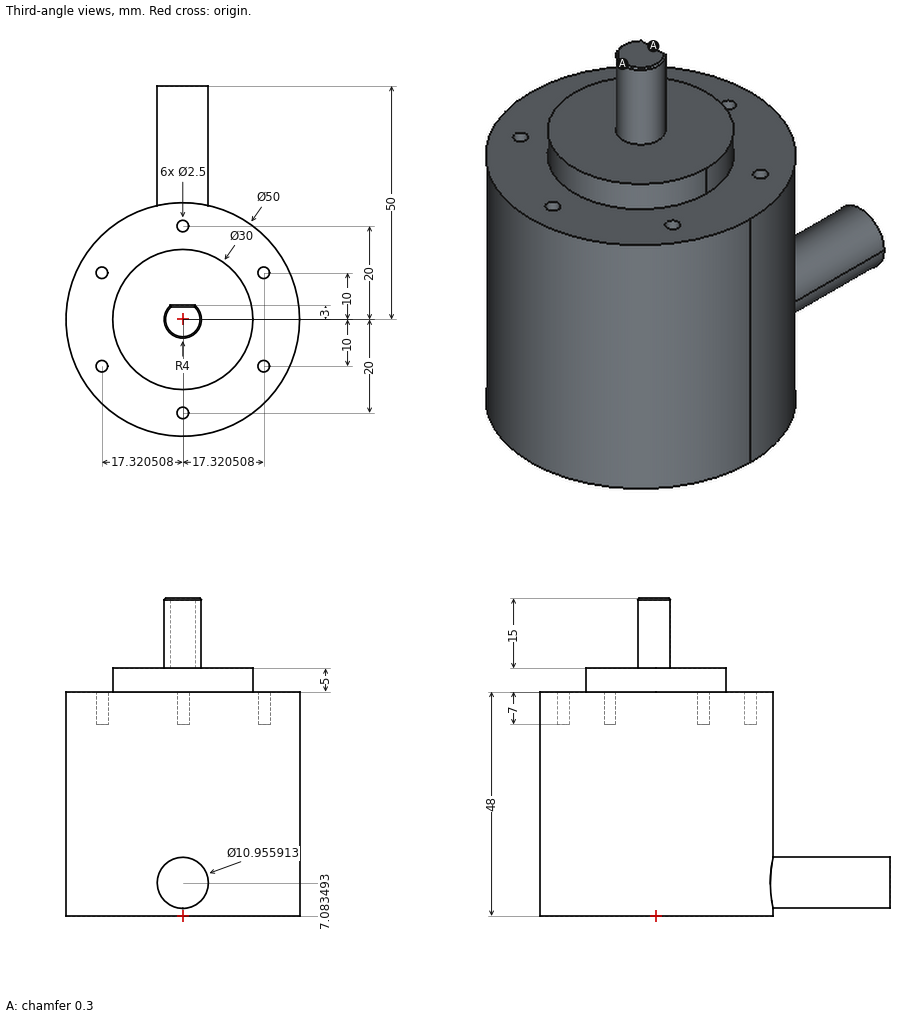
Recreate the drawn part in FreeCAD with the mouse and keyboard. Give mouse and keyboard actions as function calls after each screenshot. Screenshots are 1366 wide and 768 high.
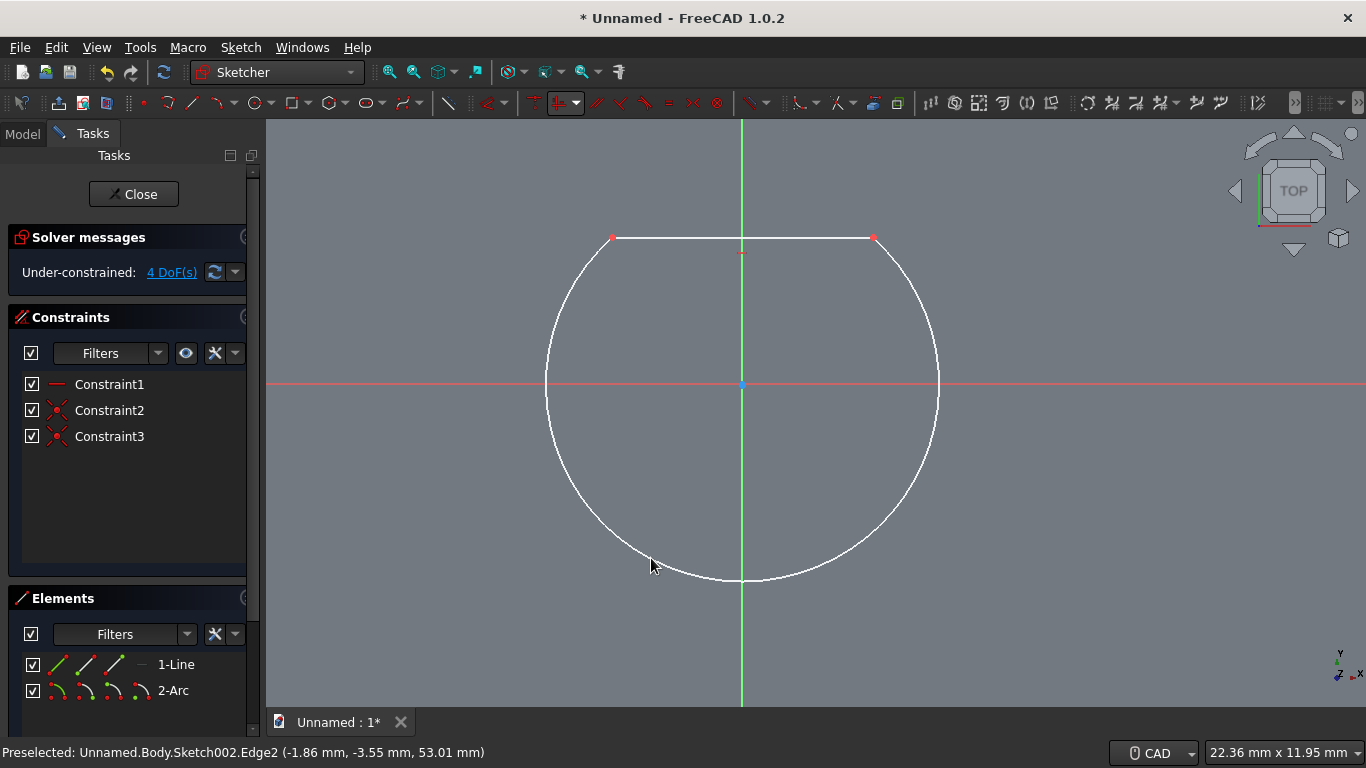
drag(732, 374, 752, 395)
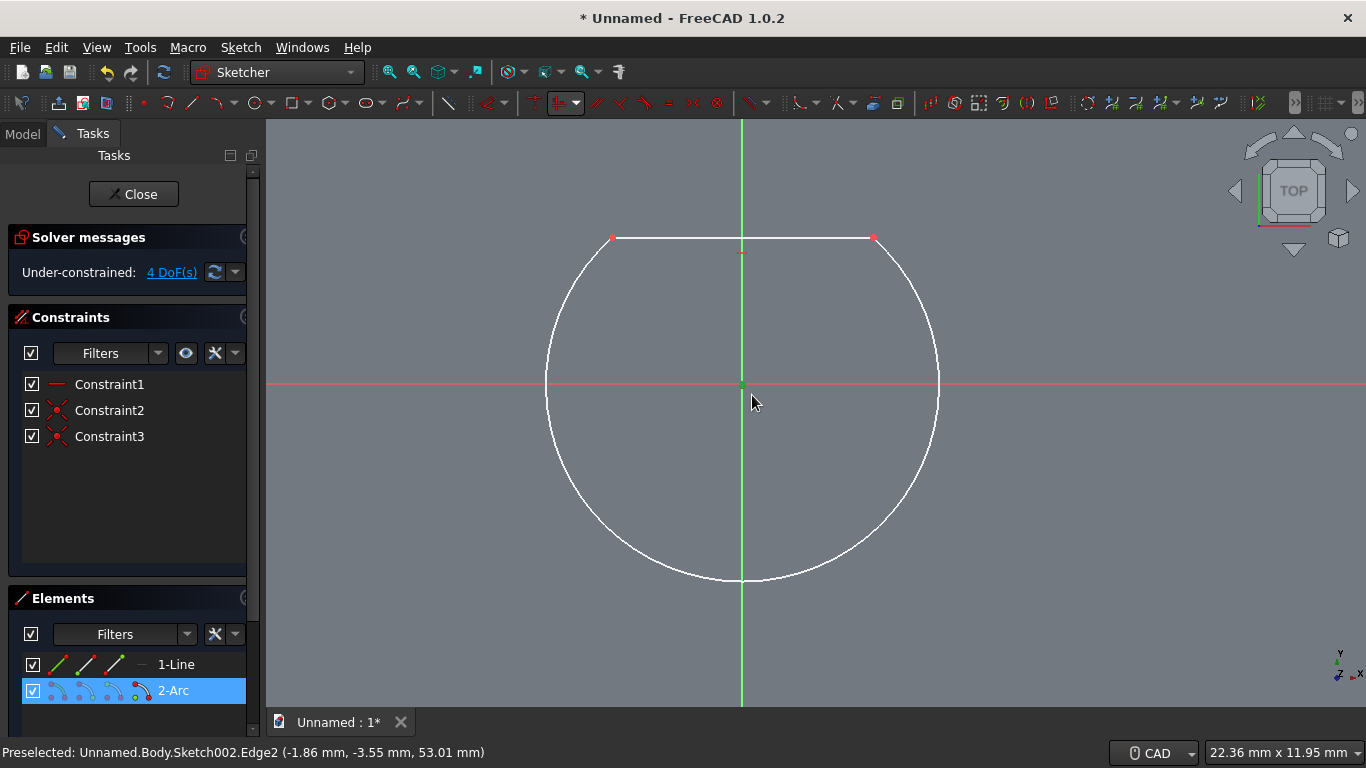
click(534, 104)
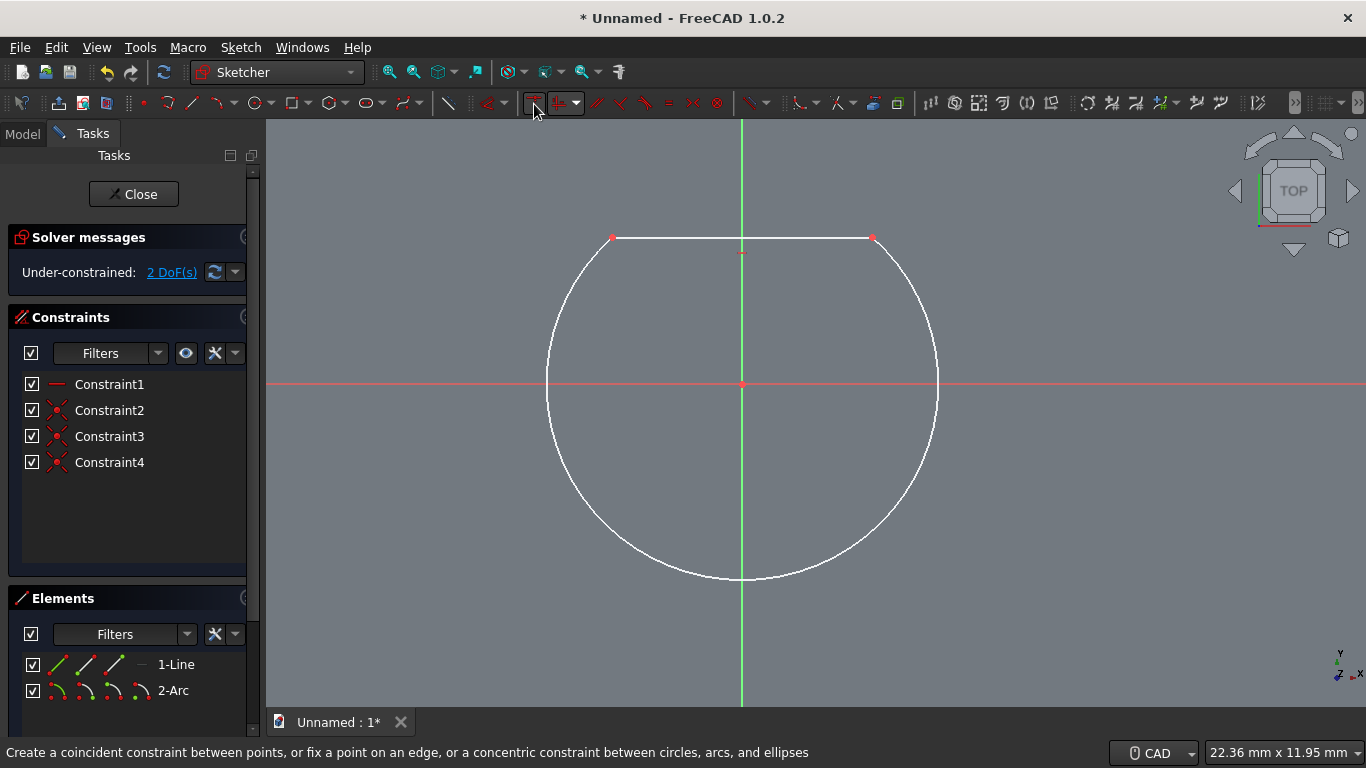
click(581, 496)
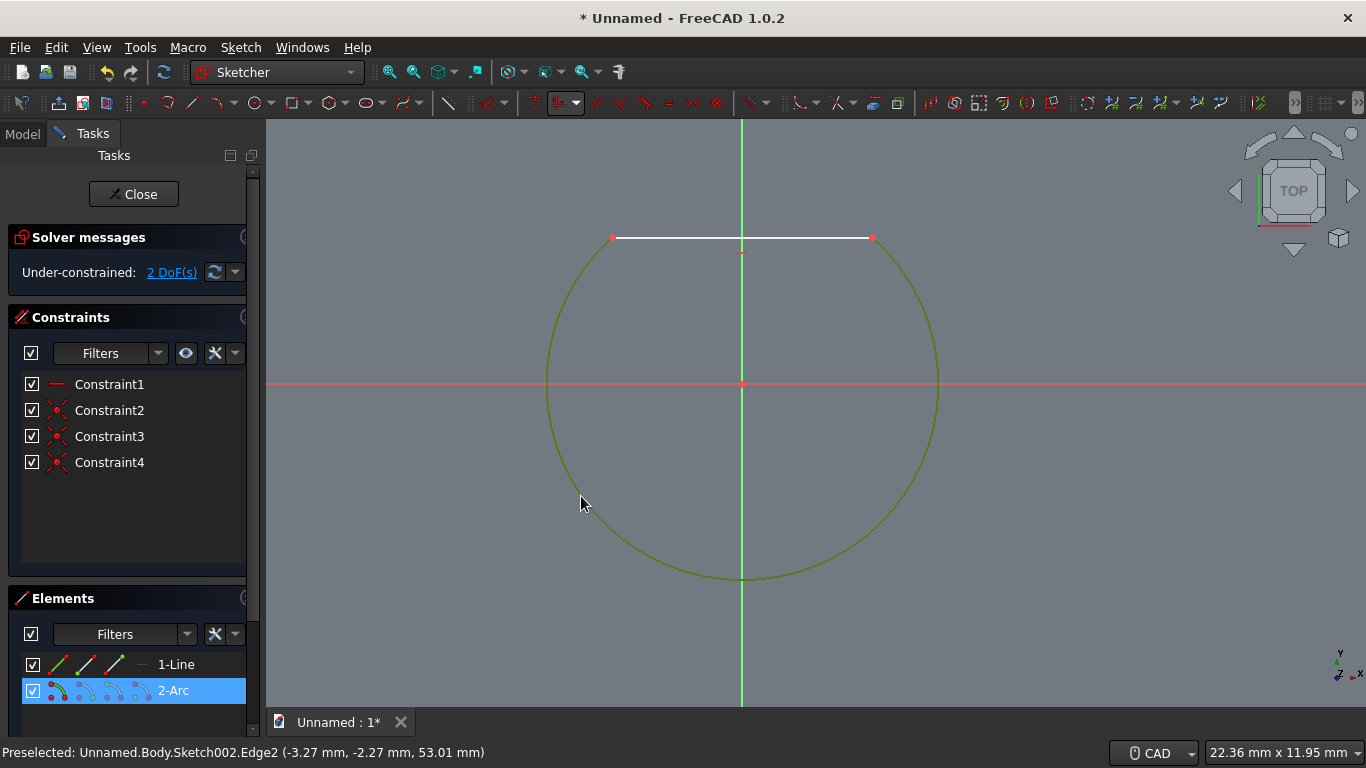
key(k)
key(r)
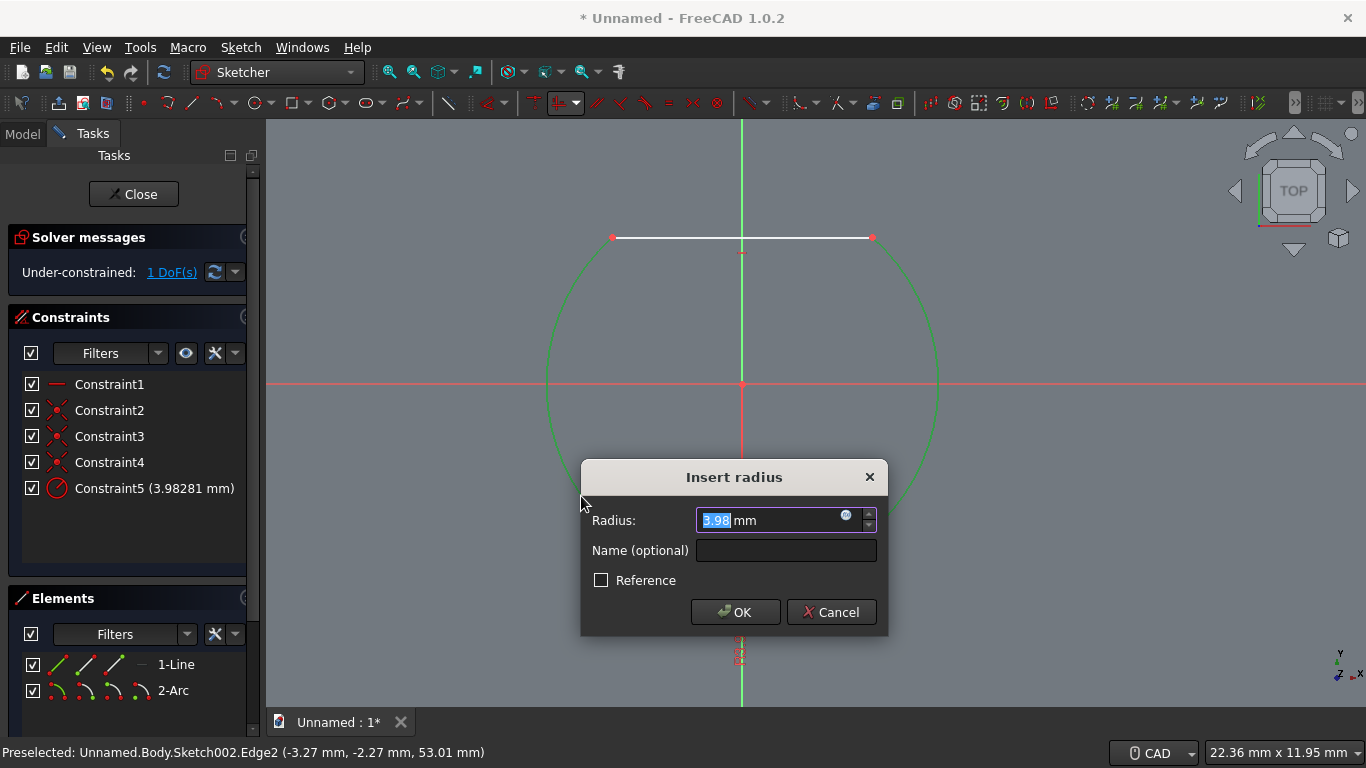
text(4)
key(Return)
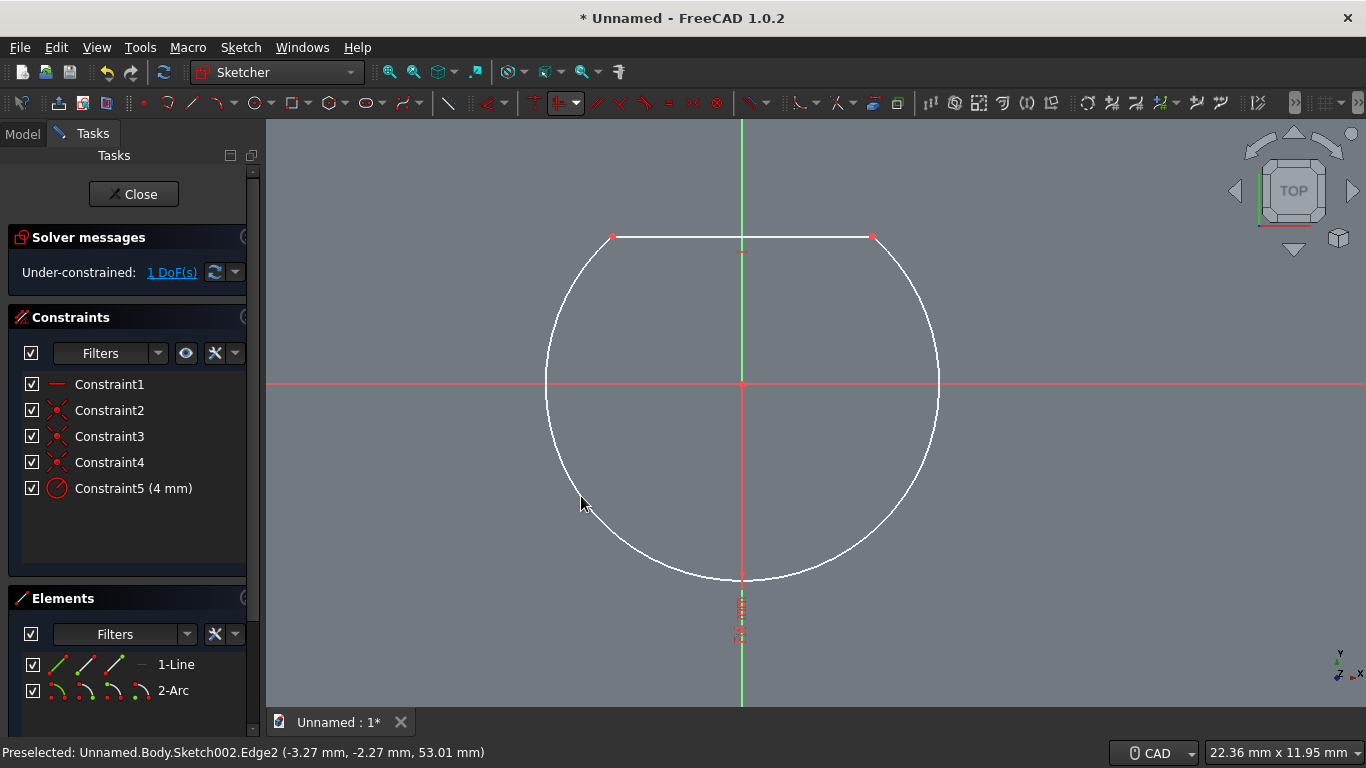
click(873, 237)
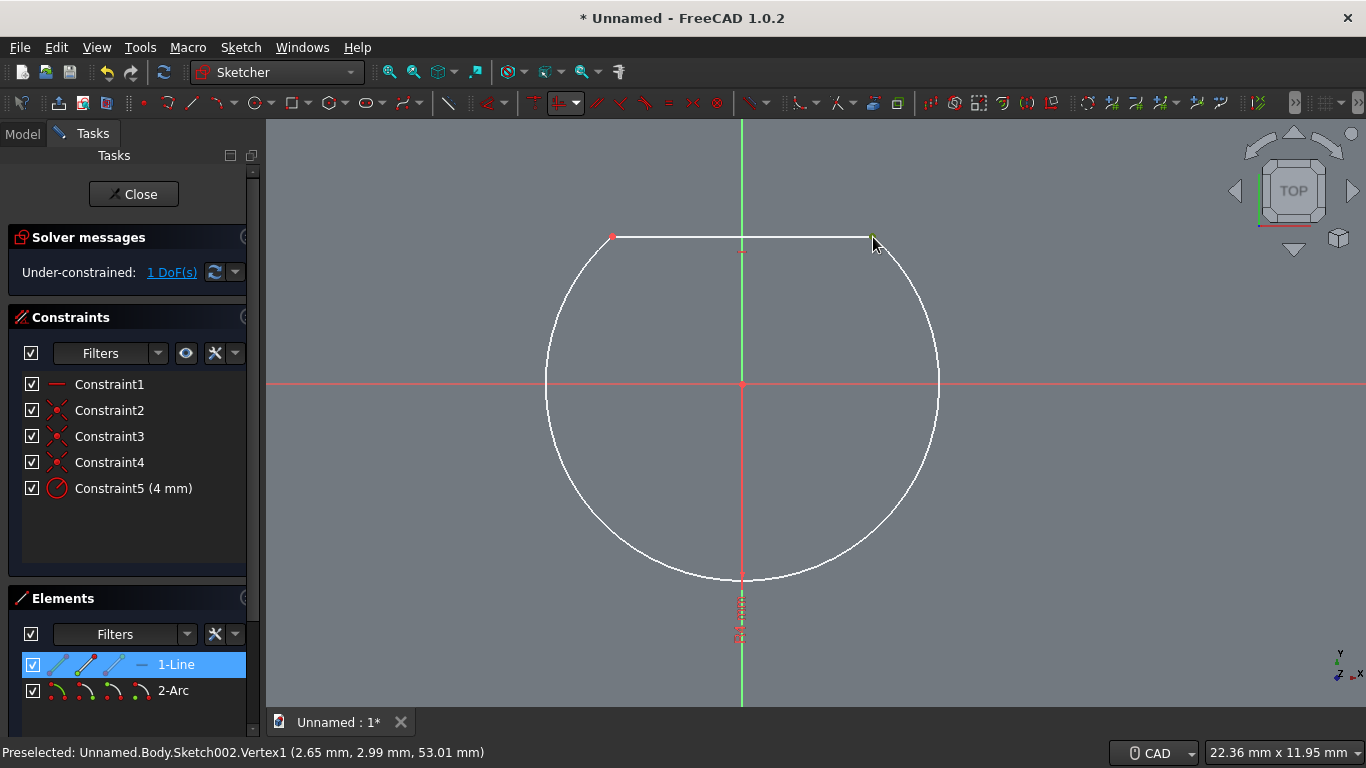
click(506, 104)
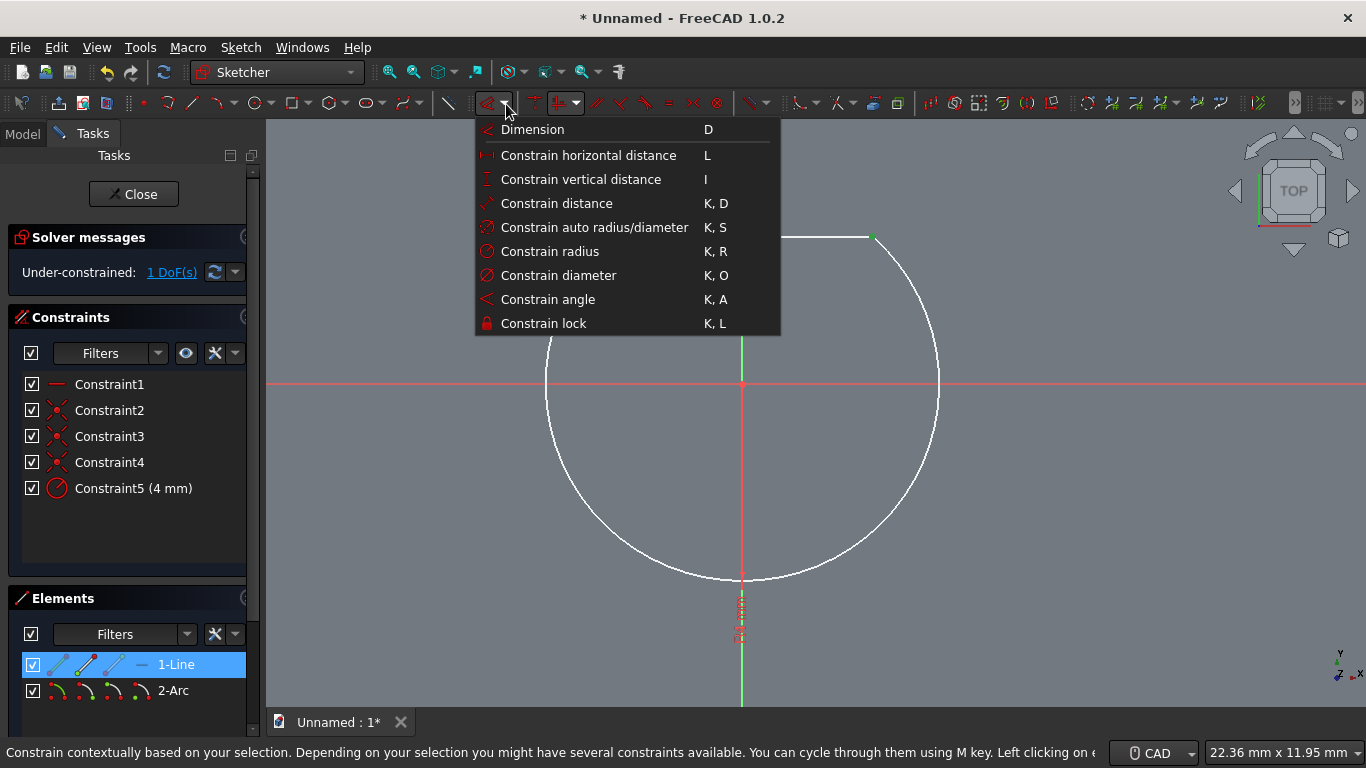
click(628, 179)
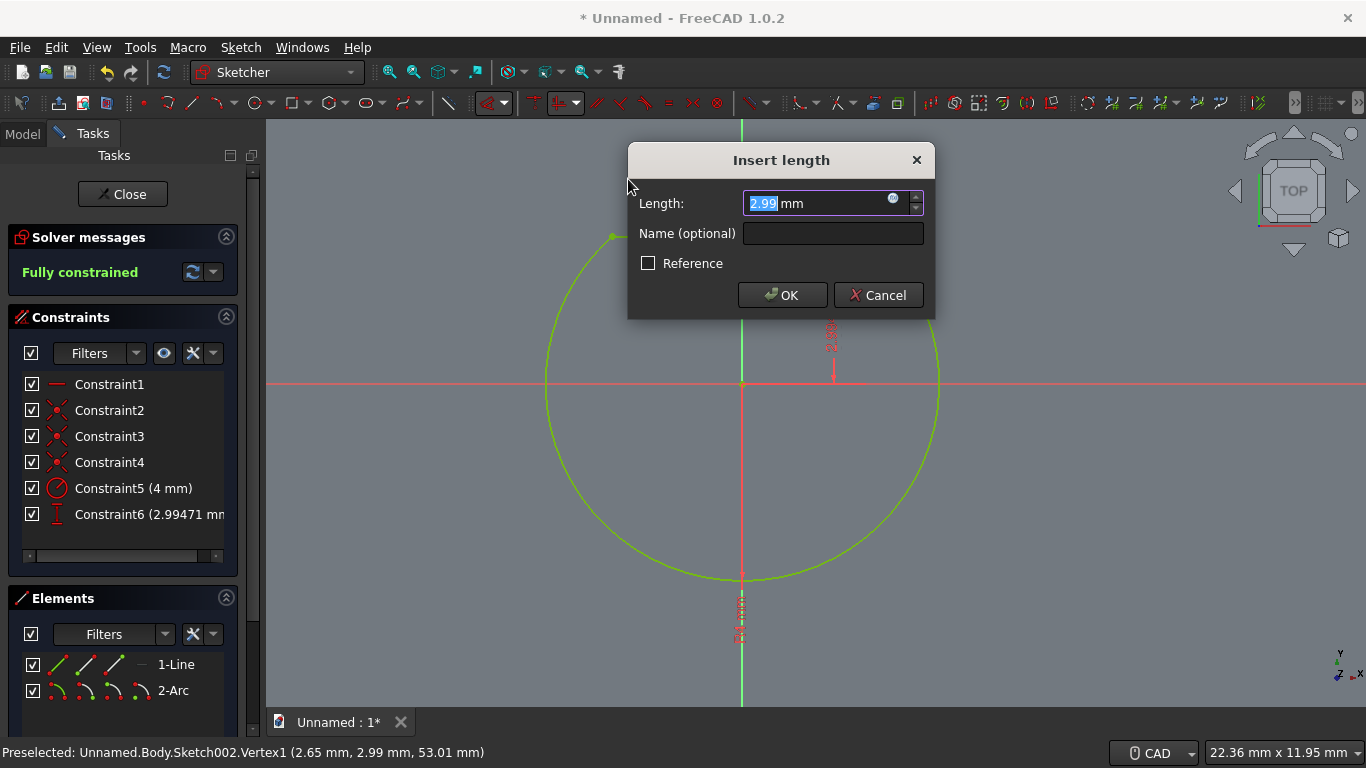
text(3)
key(Return)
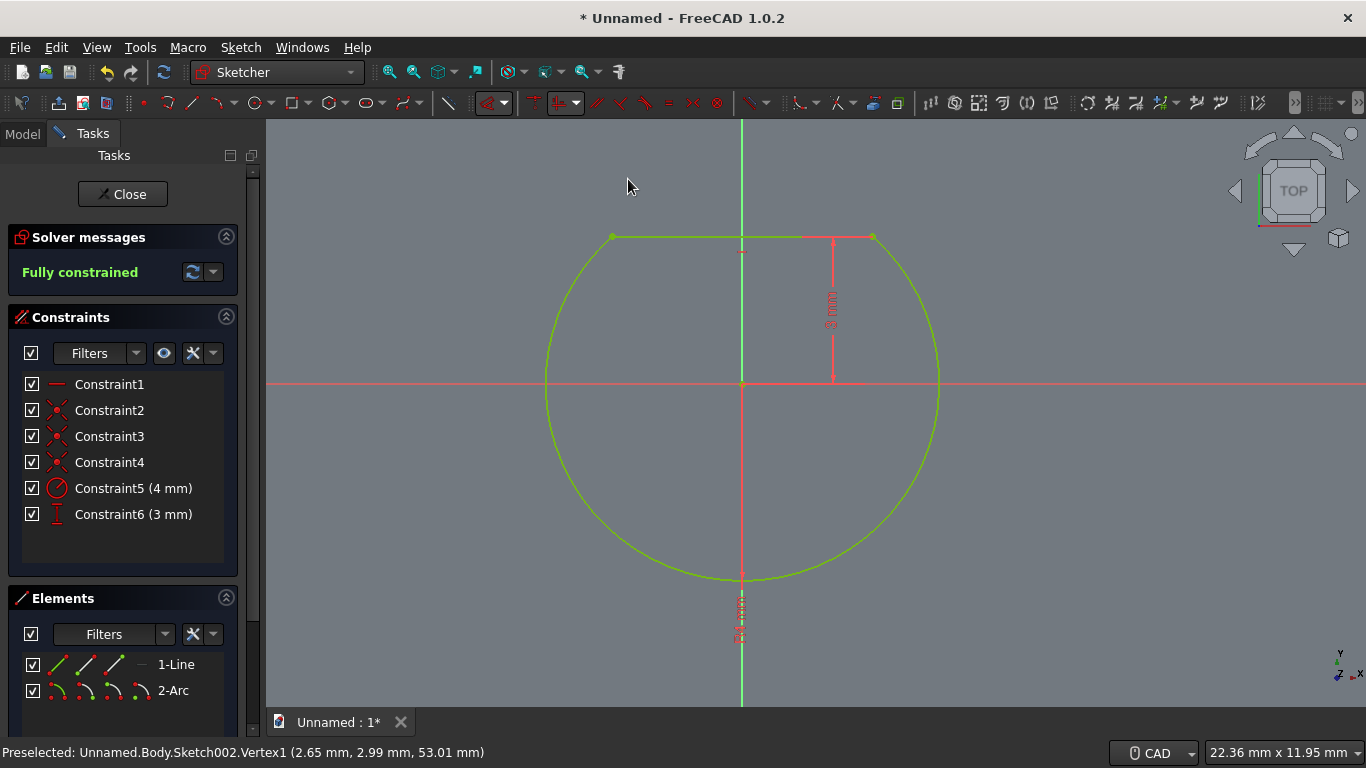
click(123, 194)